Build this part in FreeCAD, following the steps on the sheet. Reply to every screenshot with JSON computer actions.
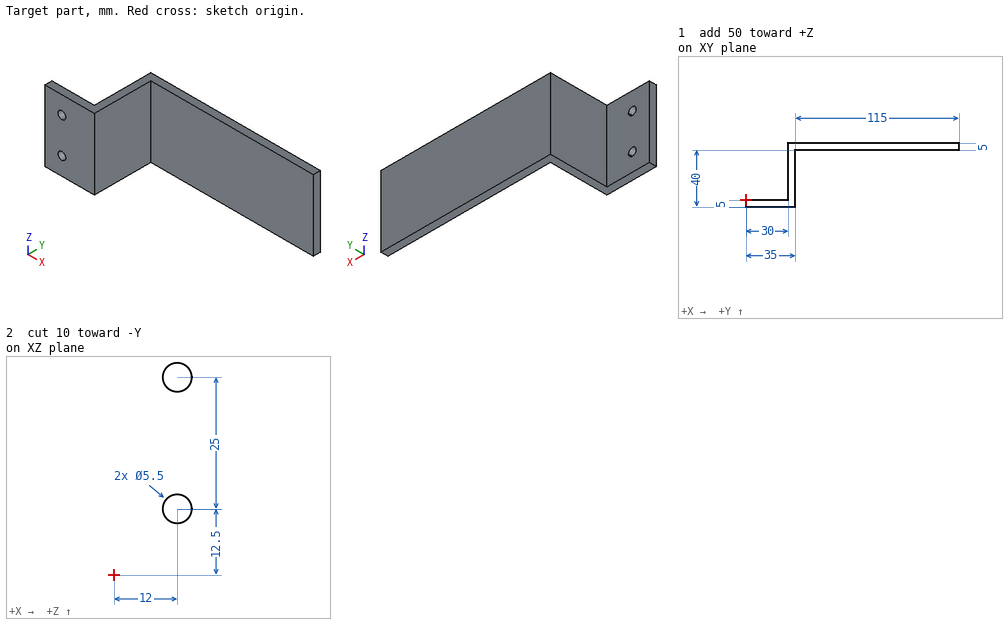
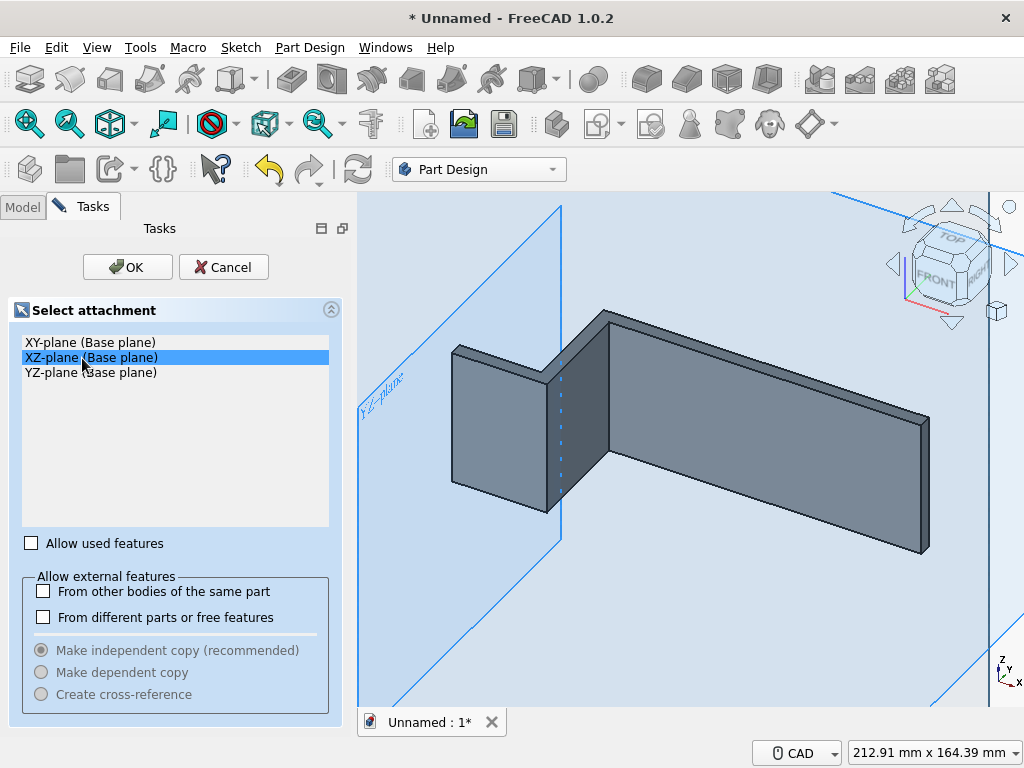
{"action": "left_click", "coordinate": [128, 267]}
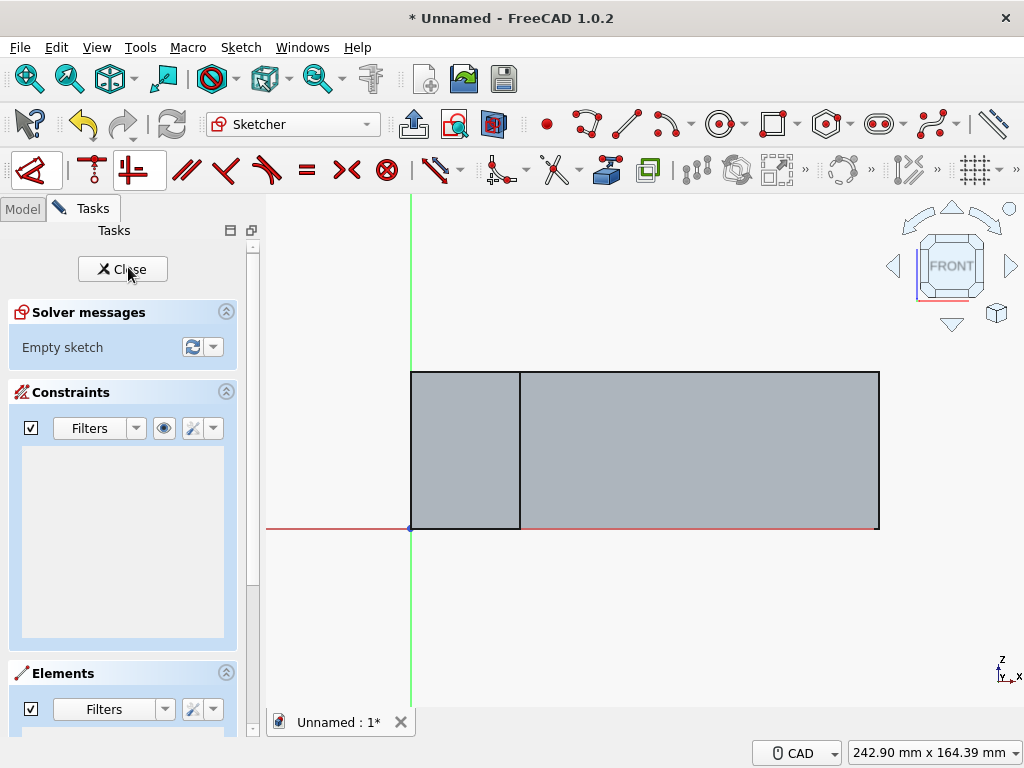
{"action": "key", "text": "q s"}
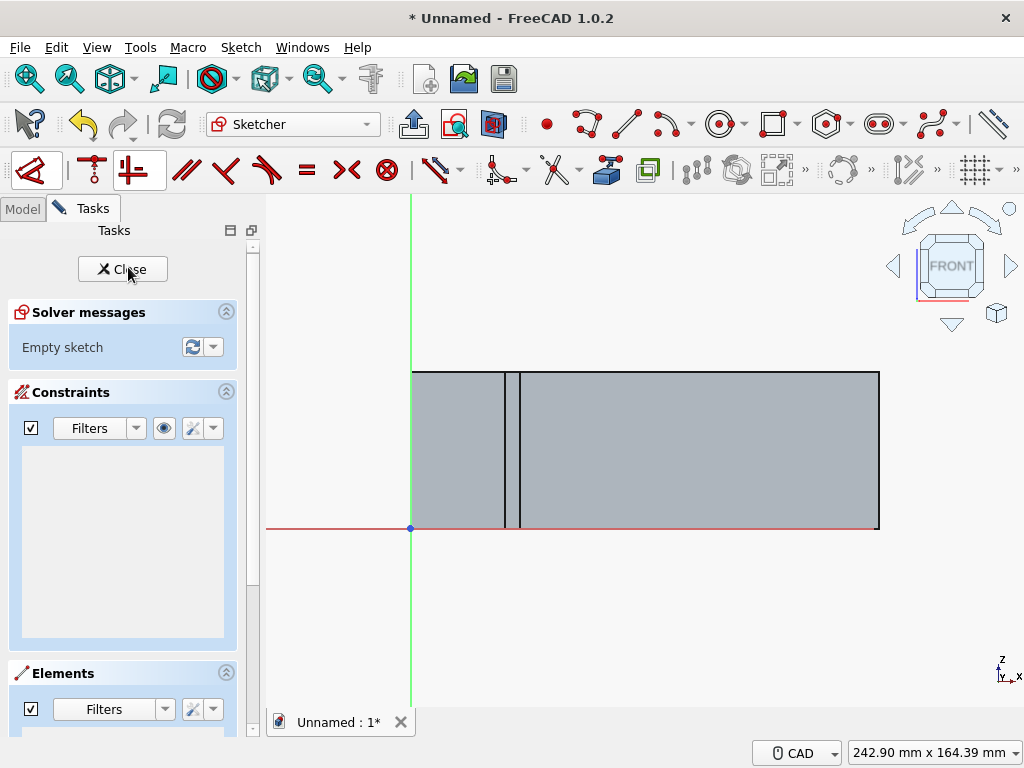
{"action": "scroll", "coordinate": [351, 475], "scroll_direction": "up", "scroll_amount": 5}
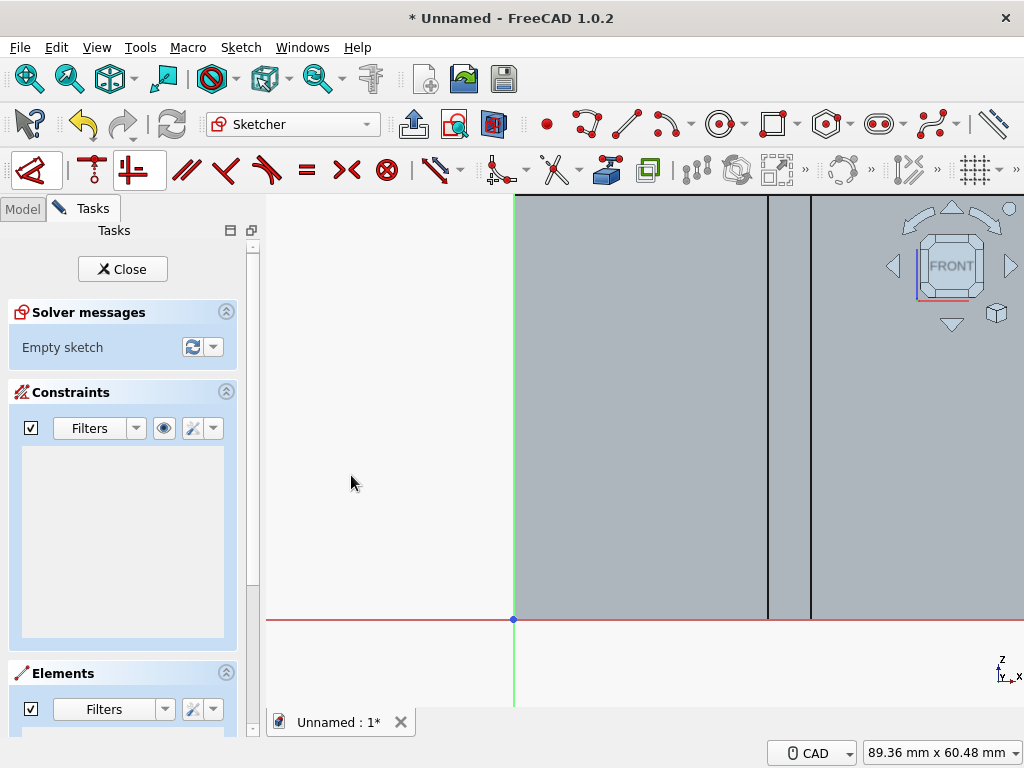
{"action": "key", "text": "g c"}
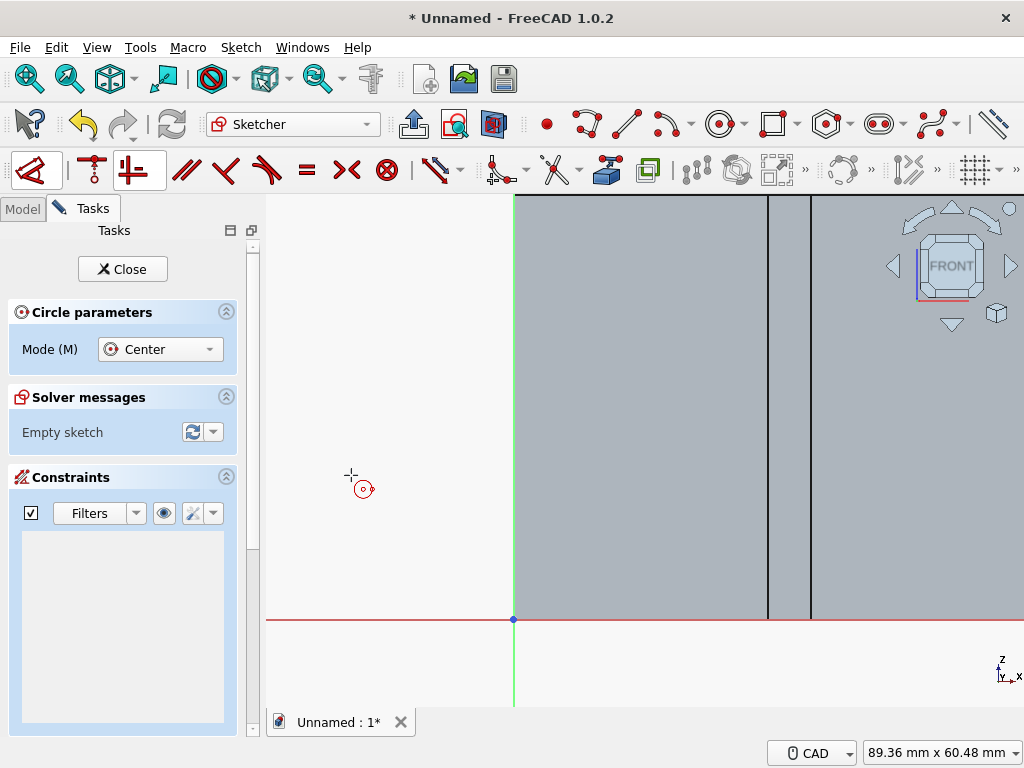
{"action": "left_click", "coordinate": [616, 513]}
{"action": "left_click", "coordinate": [632, 497]}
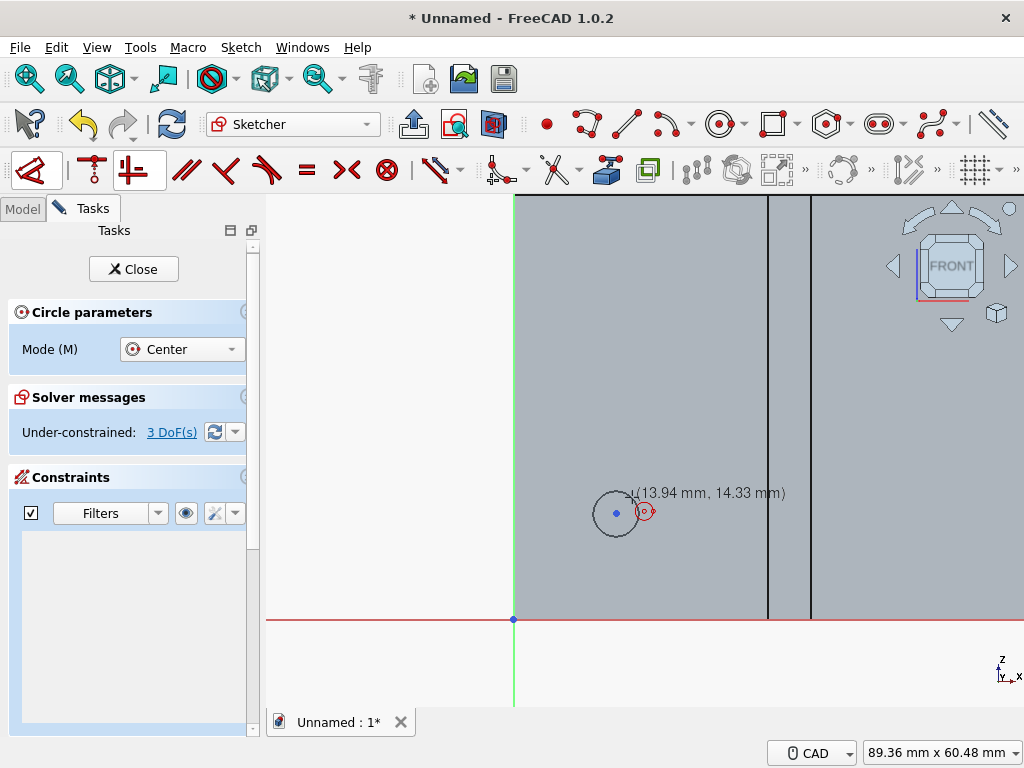
{"action": "left_click", "coordinate": [616, 301]}
{"action": "left_click", "coordinate": [632, 285]}
{"action": "key", "text": "Escape"}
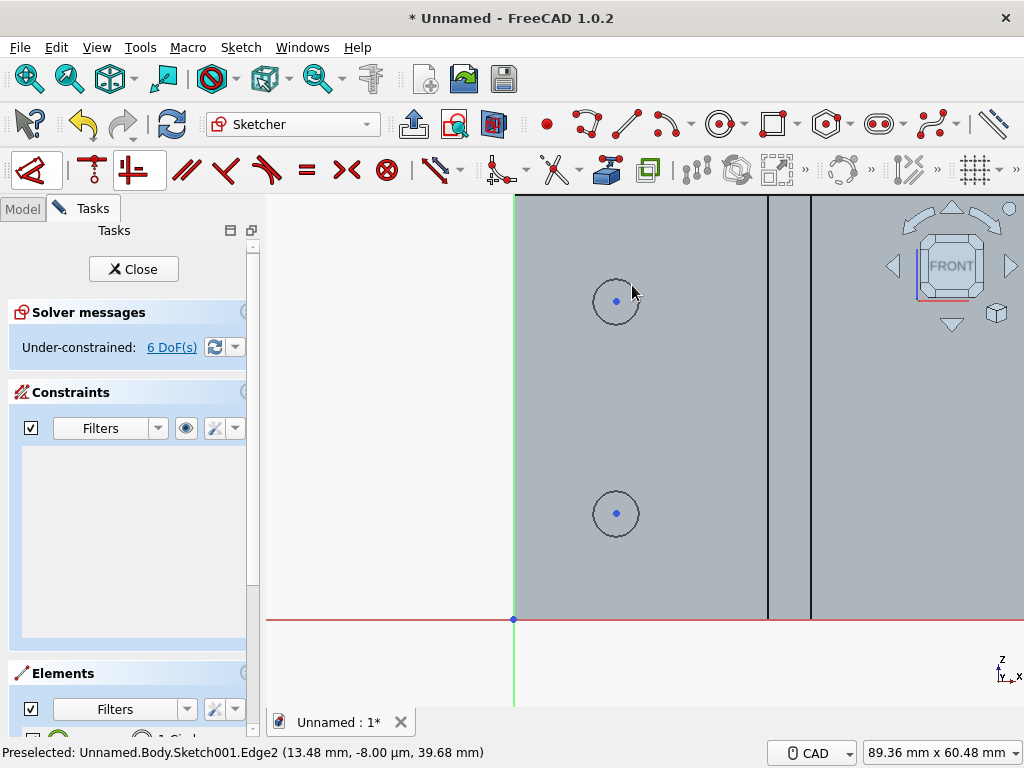
{"action": "left_click", "coordinate": [632, 498]}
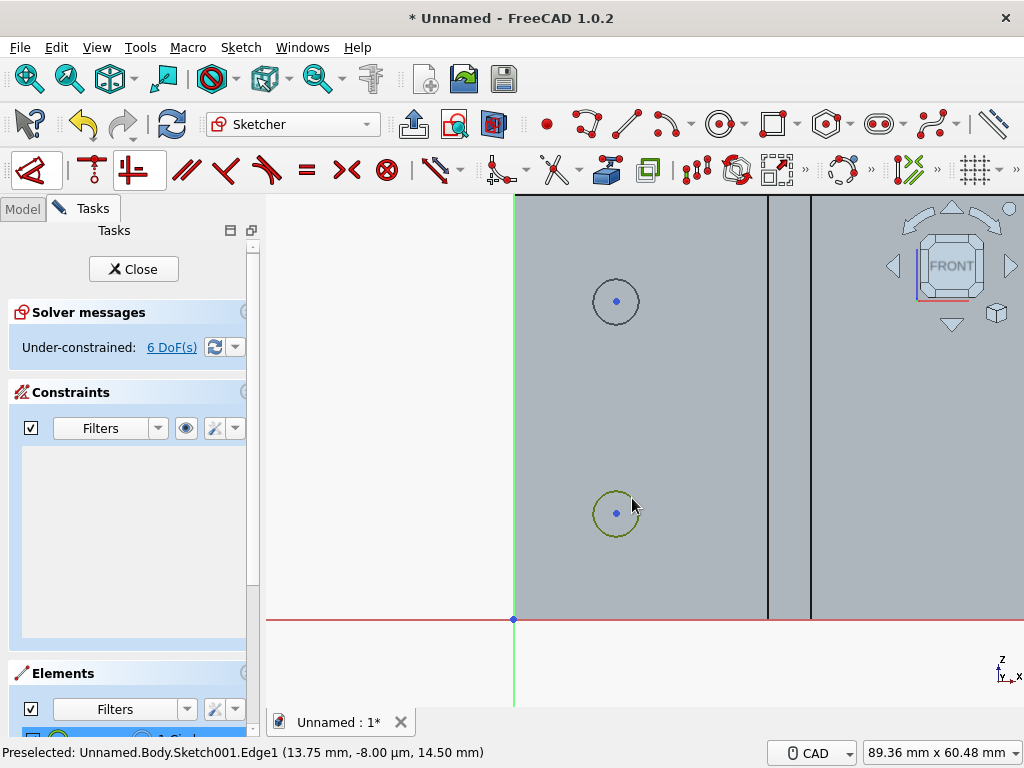
{"action": "left_click", "coordinate": [632, 286]}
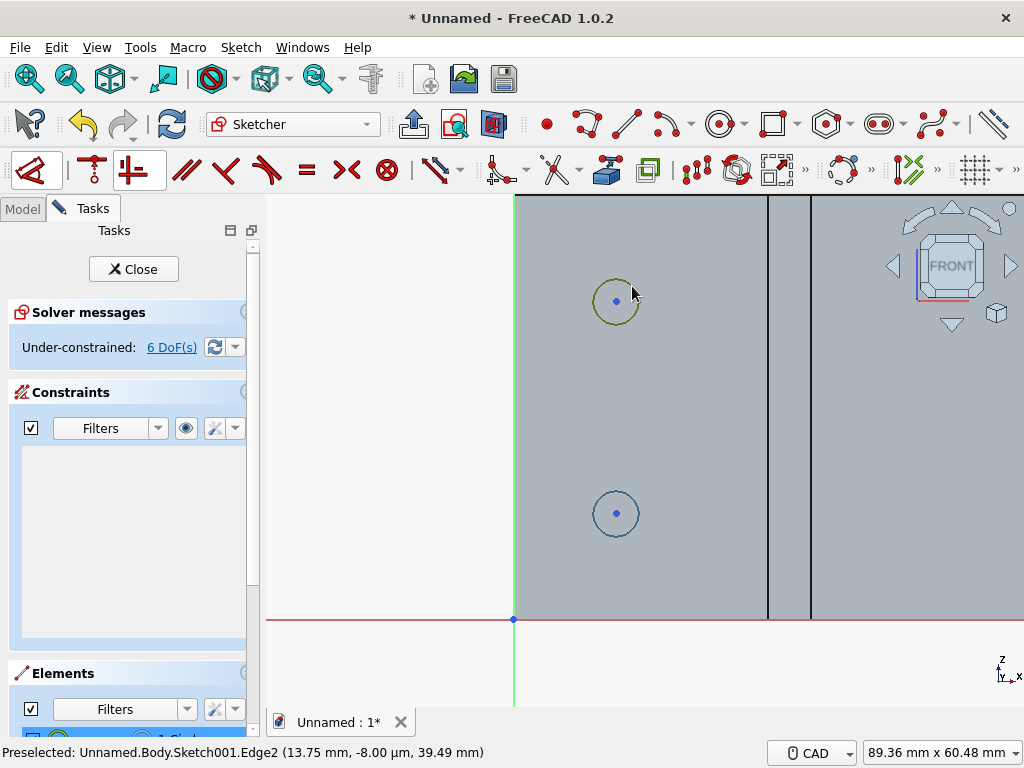
{"action": "left_click", "coordinate": [308, 170]}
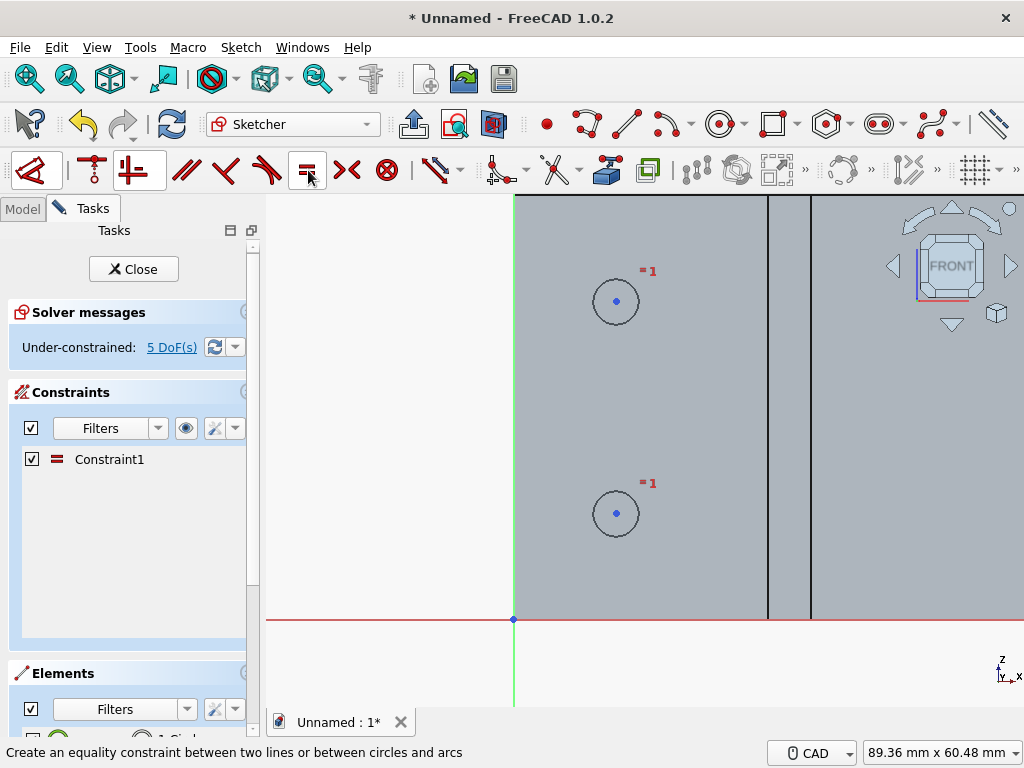
{"action": "left_click", "coordinate": [616, 514]}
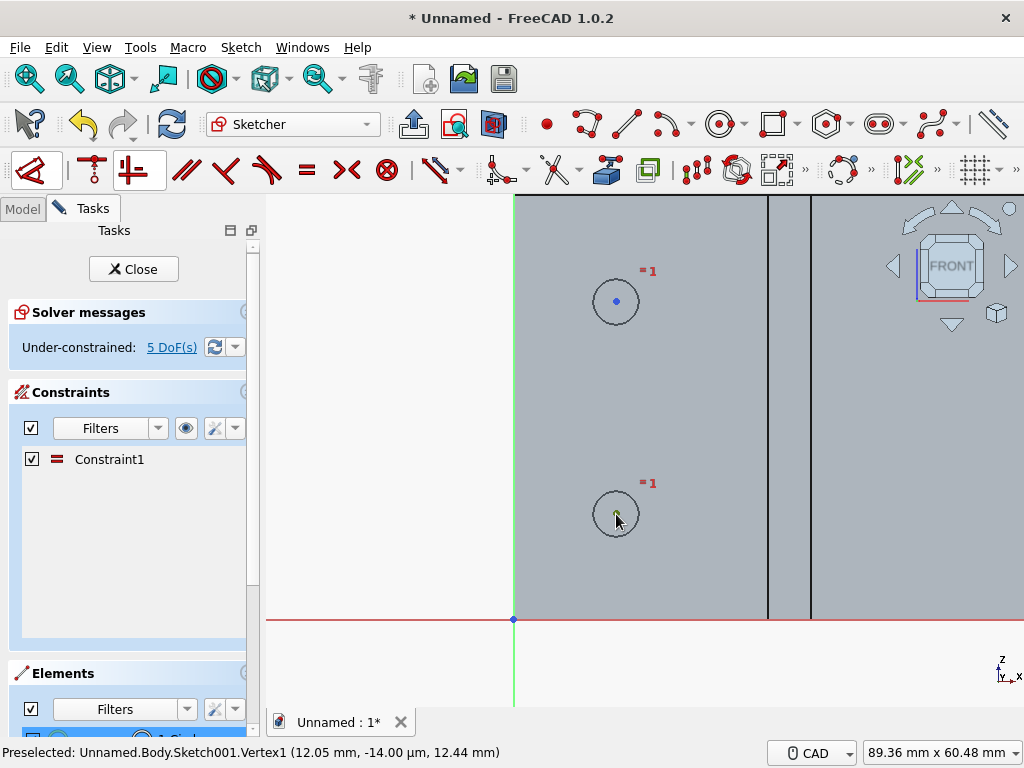
{"action": "left_click", "coordinate": [616, 302]}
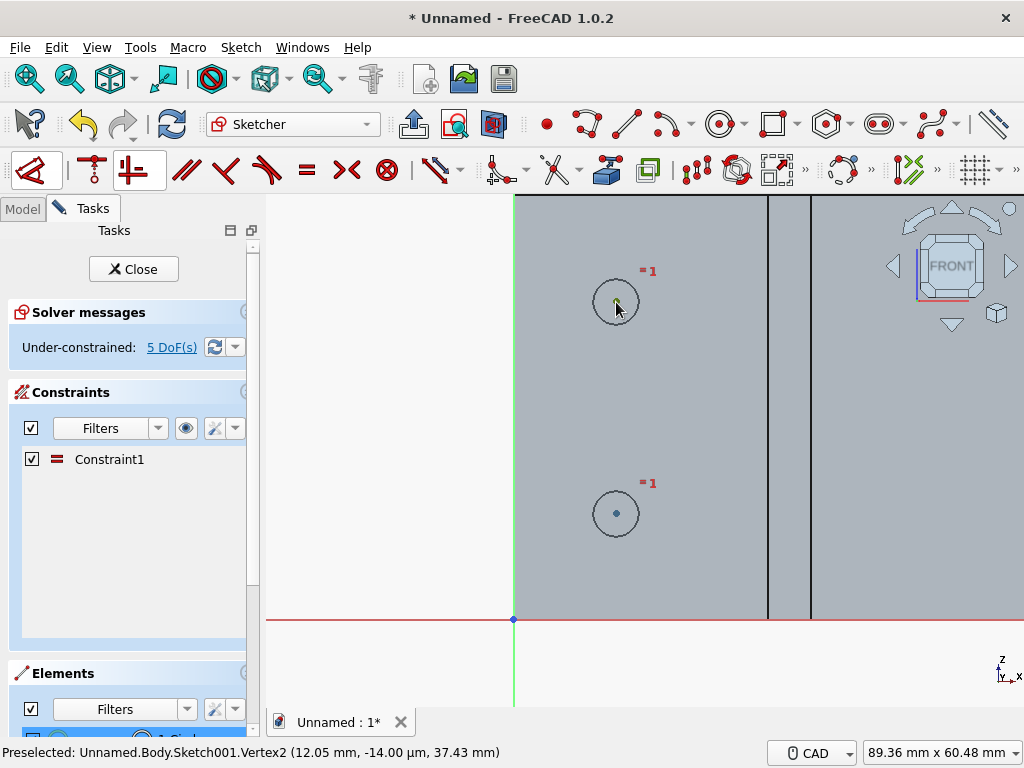
{"action": "key", "text": "v"}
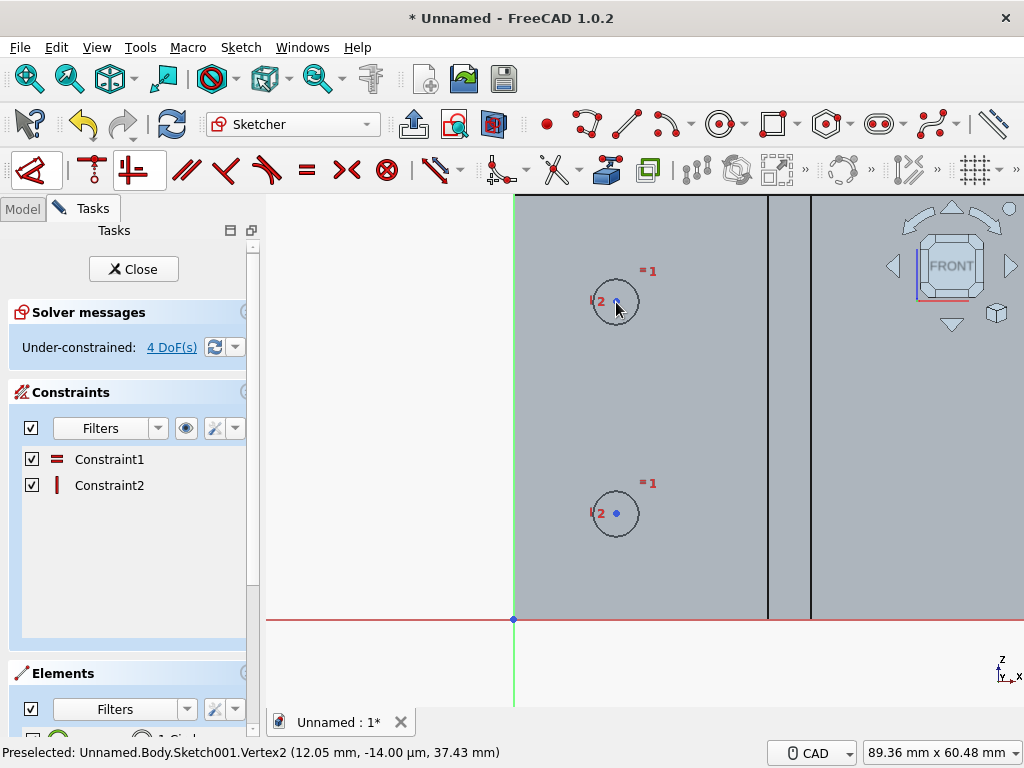
{"action": "left_click", "coordinate": [632, 498]}